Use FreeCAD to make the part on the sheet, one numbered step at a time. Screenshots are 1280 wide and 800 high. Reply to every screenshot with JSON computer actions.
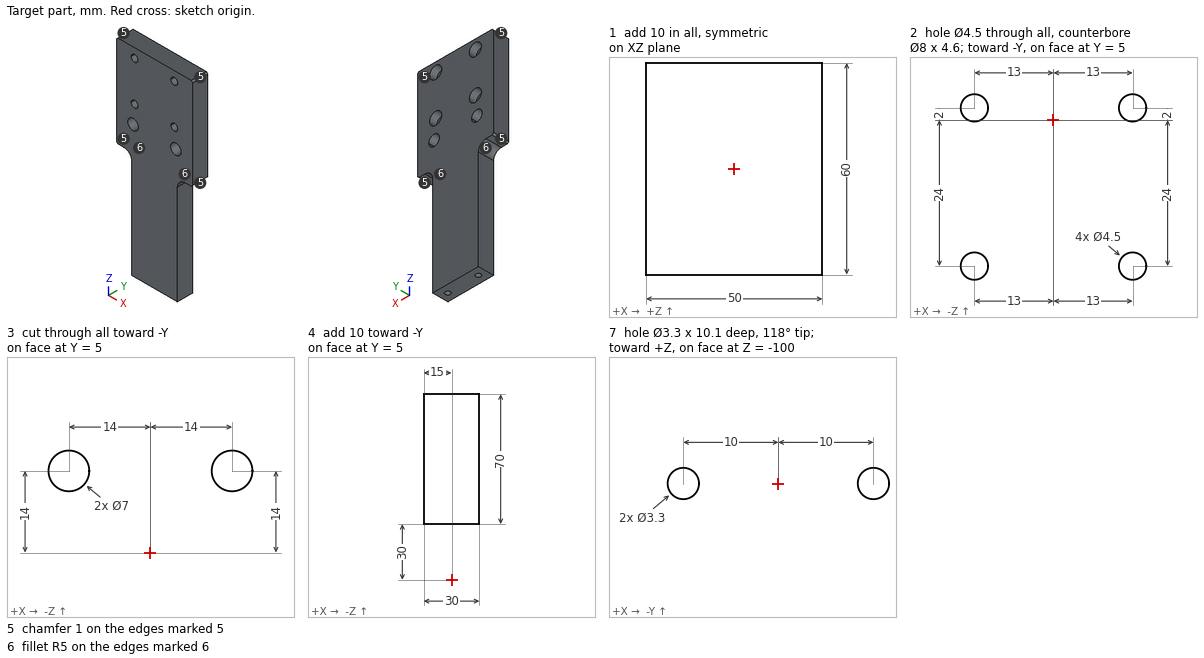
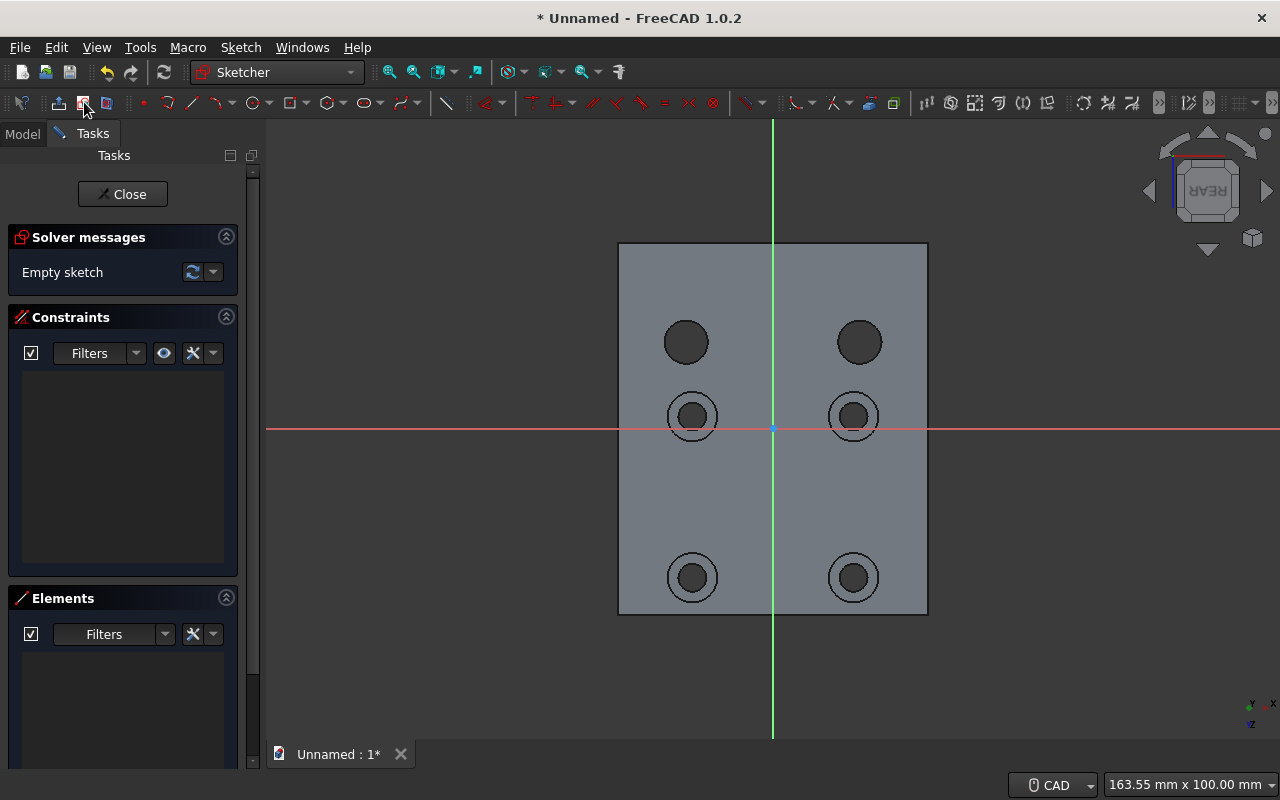
{"action": "scroll", "coordinate": [621, 711], "scroll_direction": "down", "scroll_amount": 3}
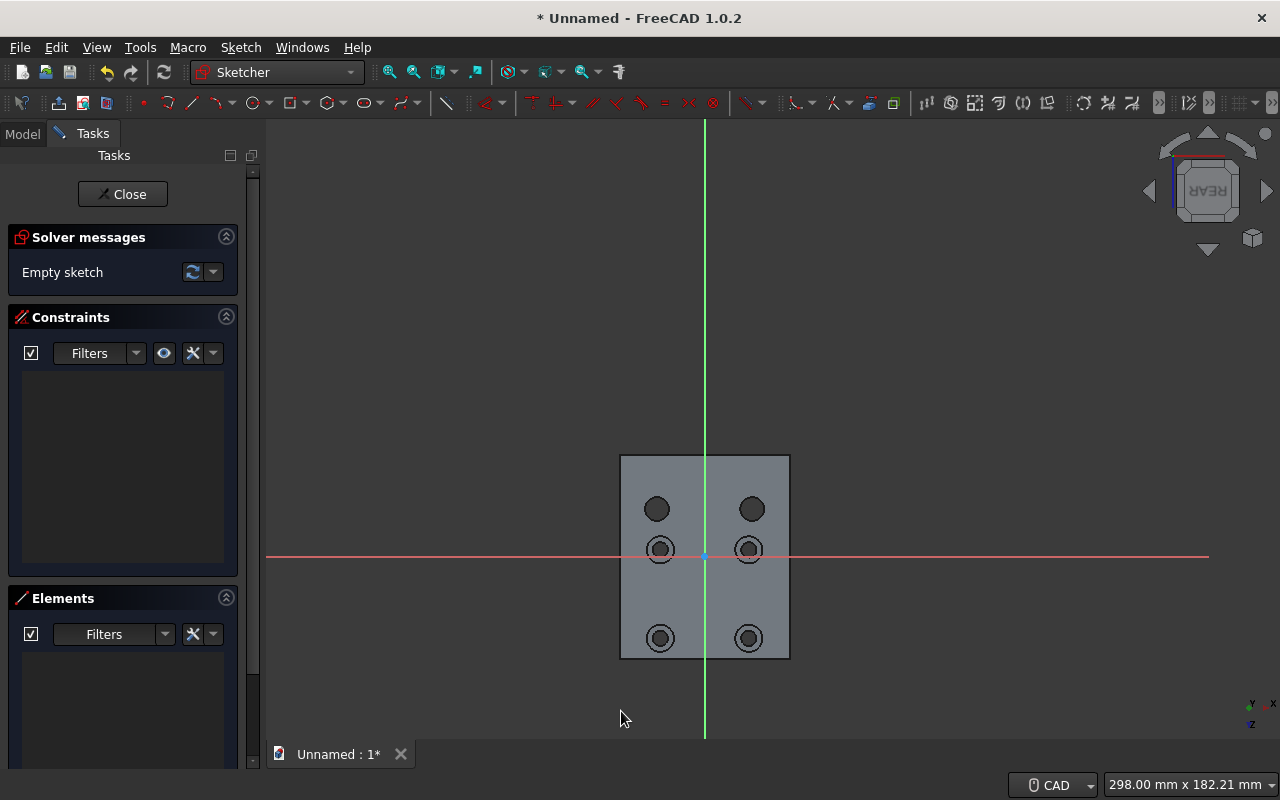
{"action": "left_click", "coordinate": [308, 104]}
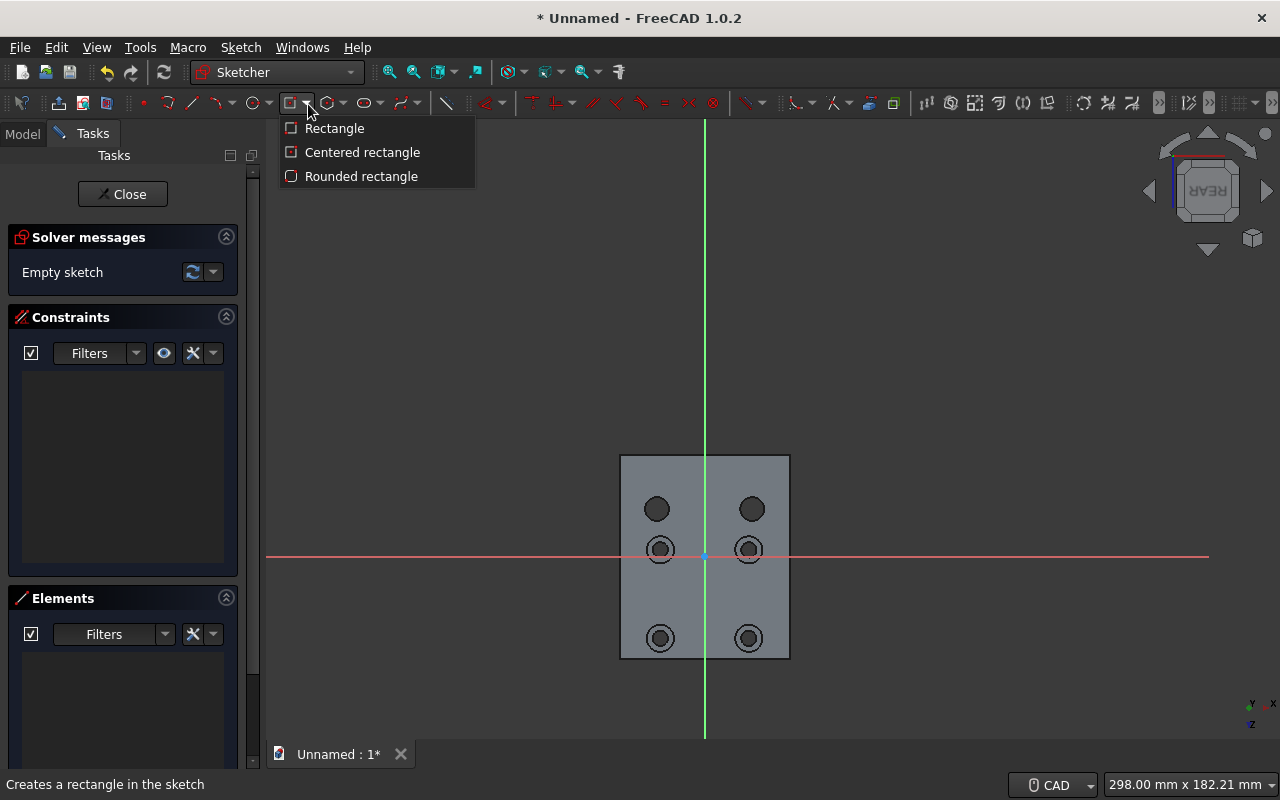
{"action": "left_click", "coordinate": [378, 128]}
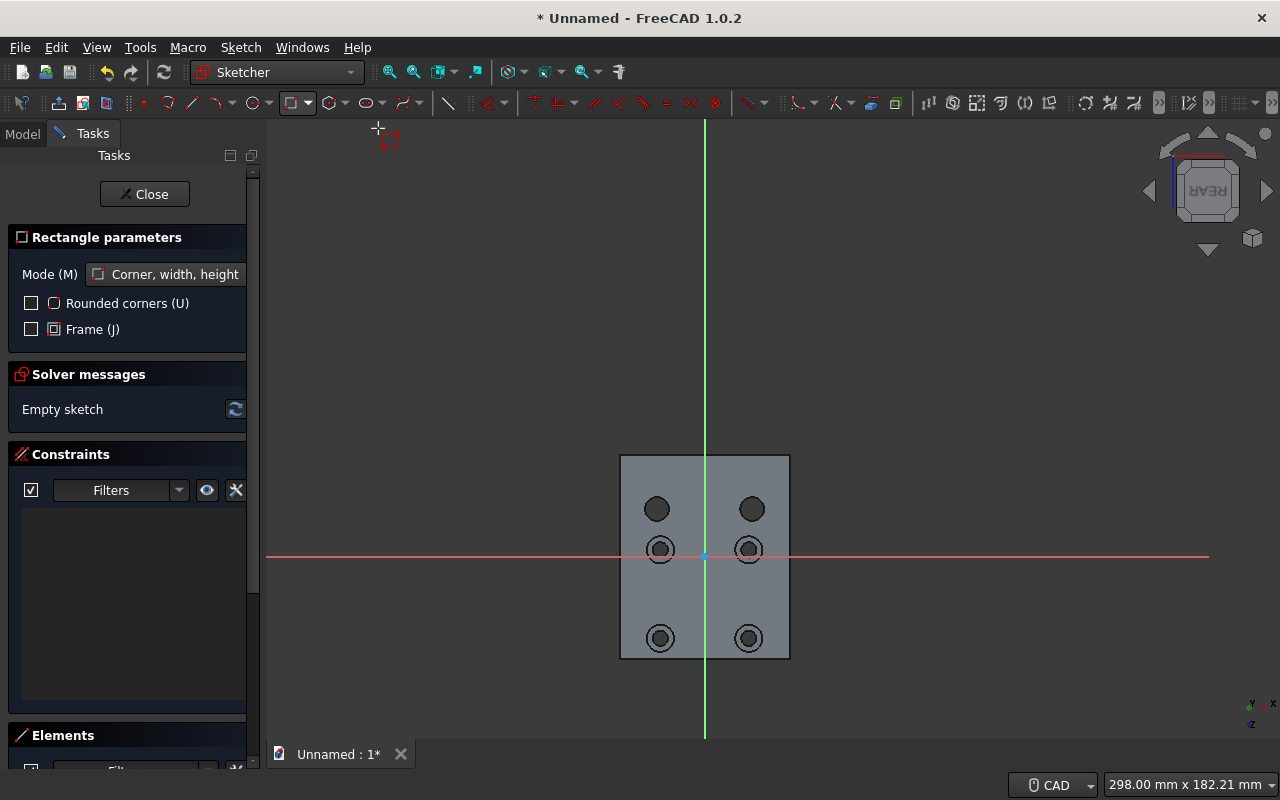
{"action": "left_click", "coordinate": [654, 216]}
{"action": "mouse_move", "coordinate": [756, 455]}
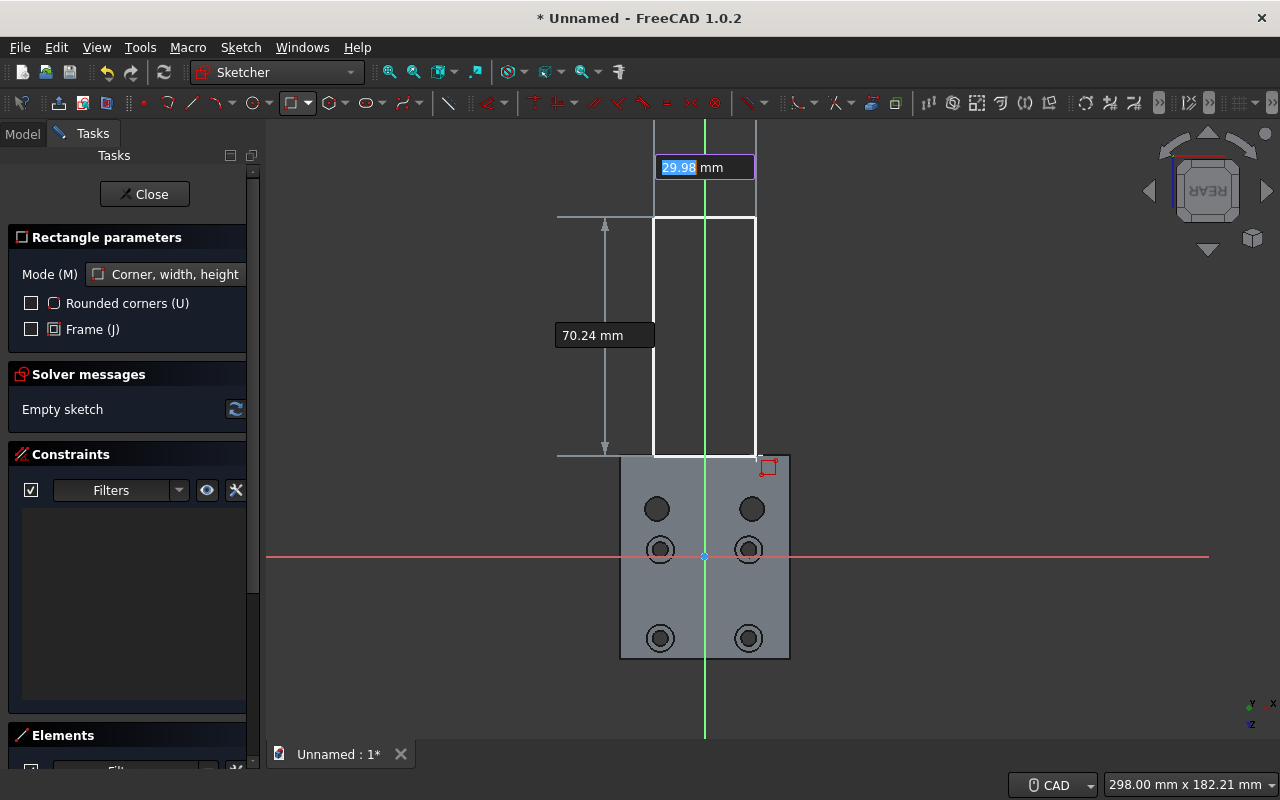
{"action": "type", "text": "30"}
{"action": "key", "text": "Tab"}
{"action": "type", "text": "70"}
{"action": "key", "text": "Return"}
{"action": "key", "text": "Escape"}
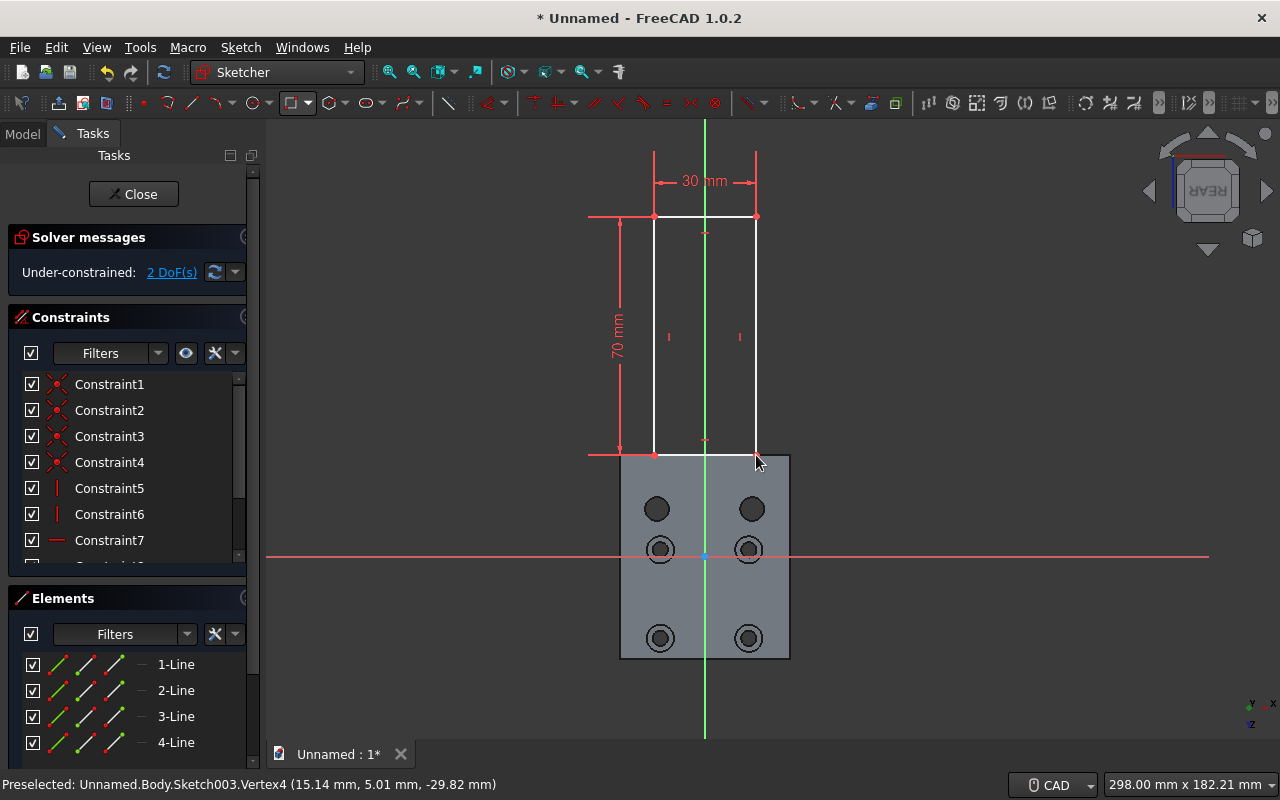
{"action": "left_click", "coordinate": [488, 104]}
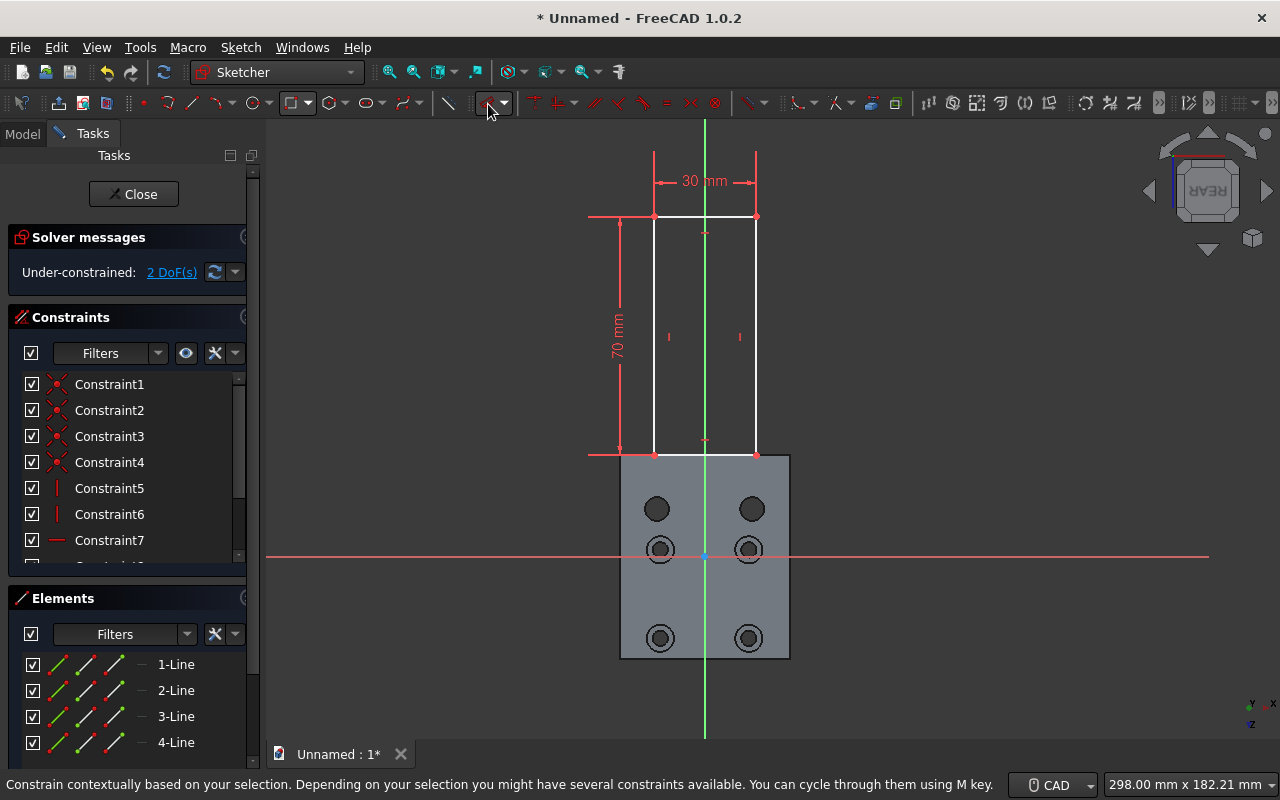
{"action": "left_click", "coordinate": [654, 217]}
{"action": "left_click", "coordinate": [679, 591]}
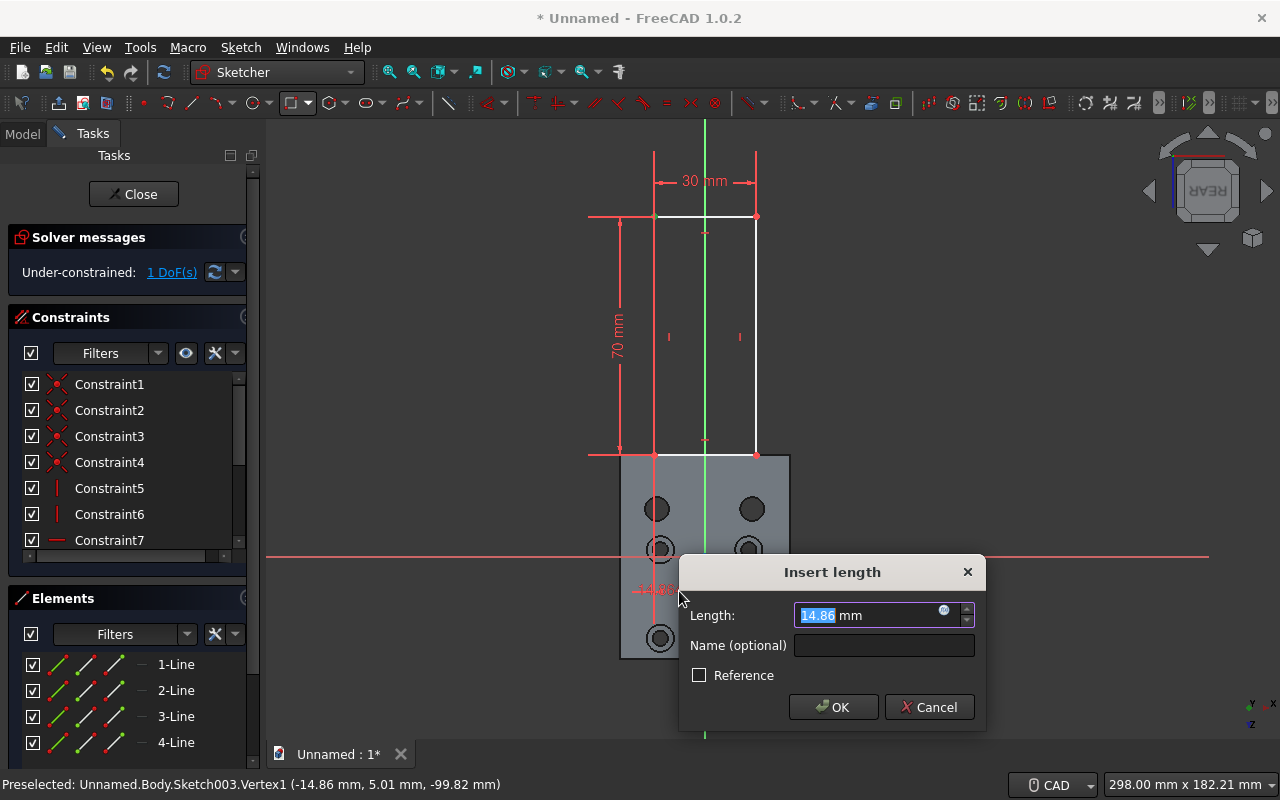
{"action": "type", "text": "15"}
{"action": "key", "text": "Return"}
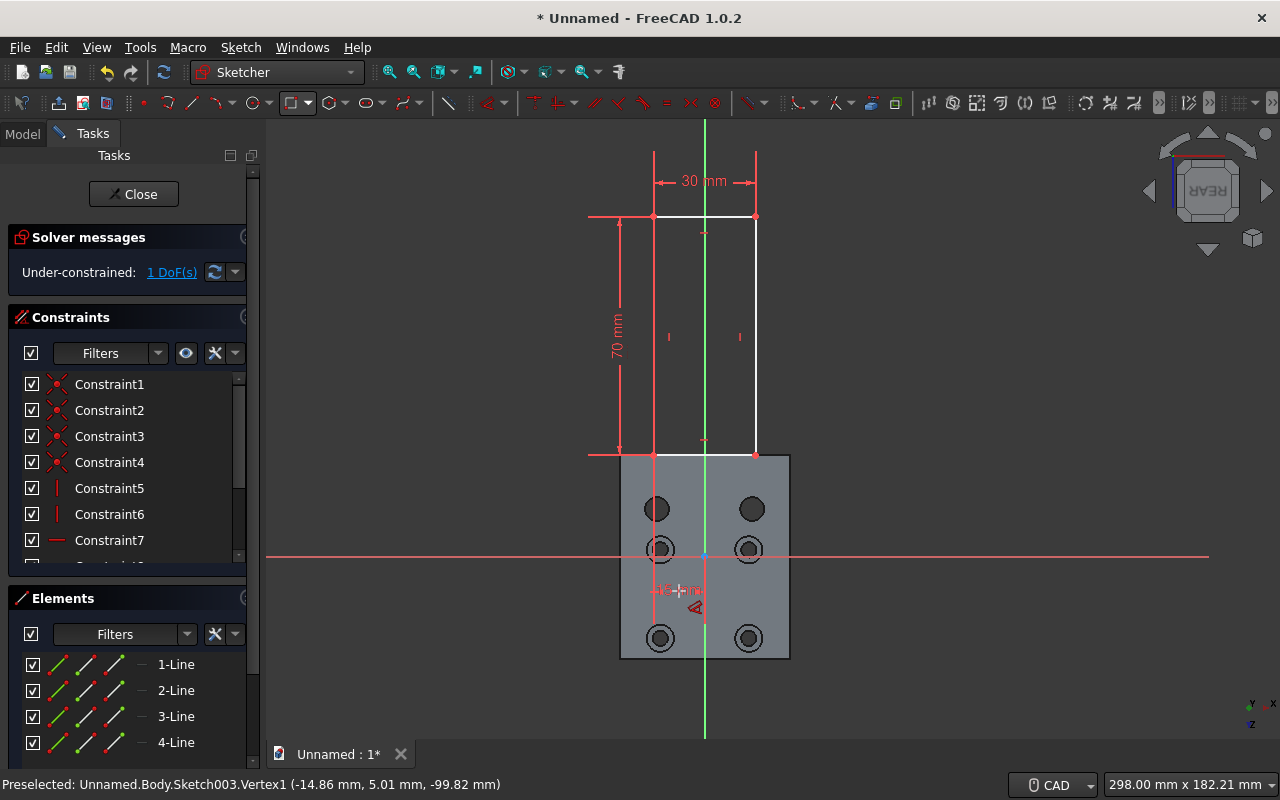
{"action": "left_click", "coordinate": [654, 455]}
{"action": "left_click", "coordinate": [620, 506]}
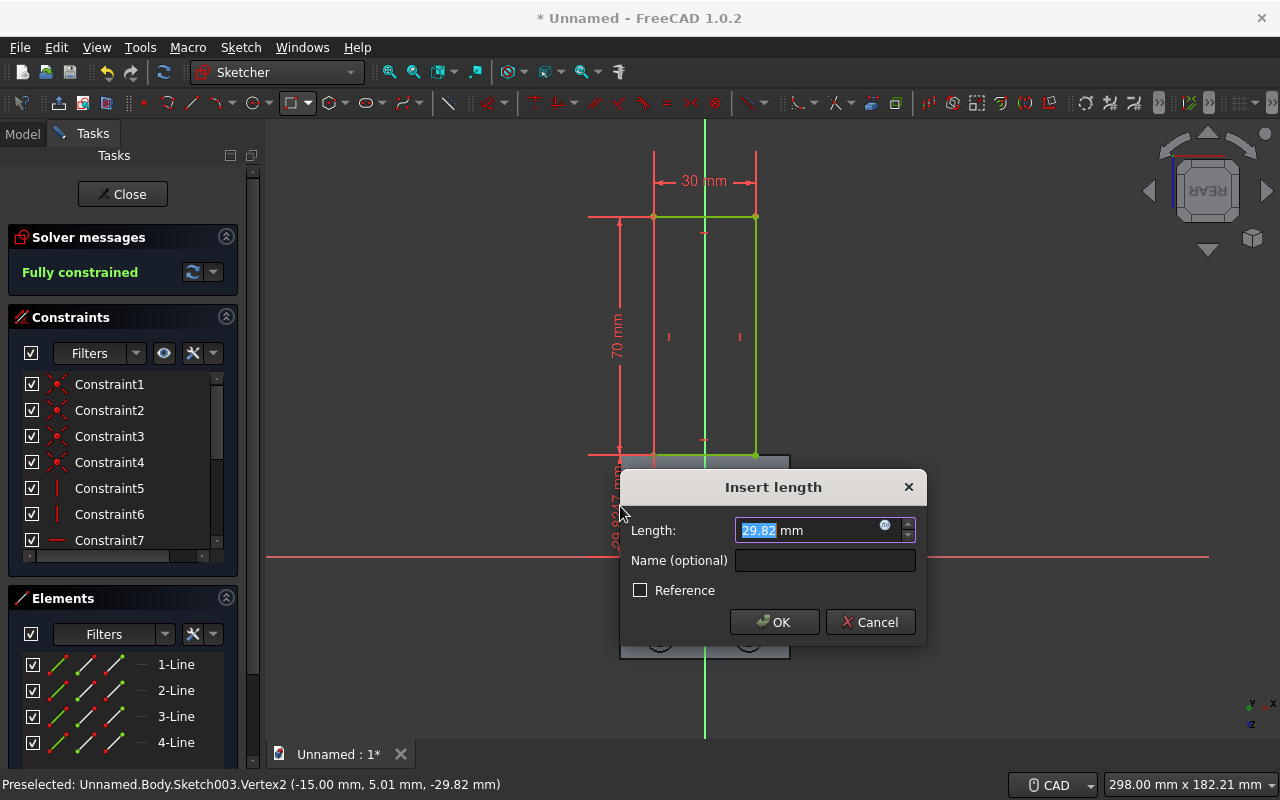
{"action": "type", "text": "30"}
{"action": "key", "text": "Return"}
{"action": "key", "text": "Escape"}